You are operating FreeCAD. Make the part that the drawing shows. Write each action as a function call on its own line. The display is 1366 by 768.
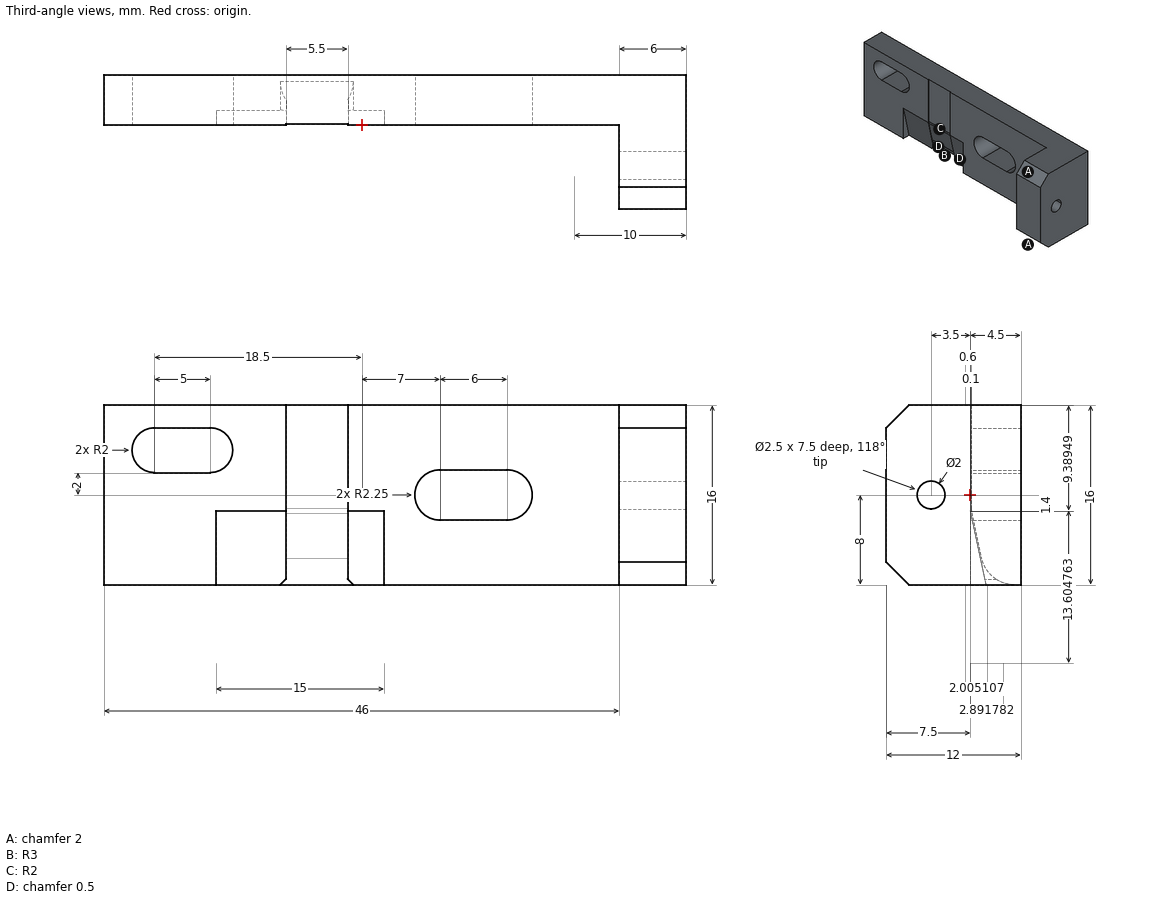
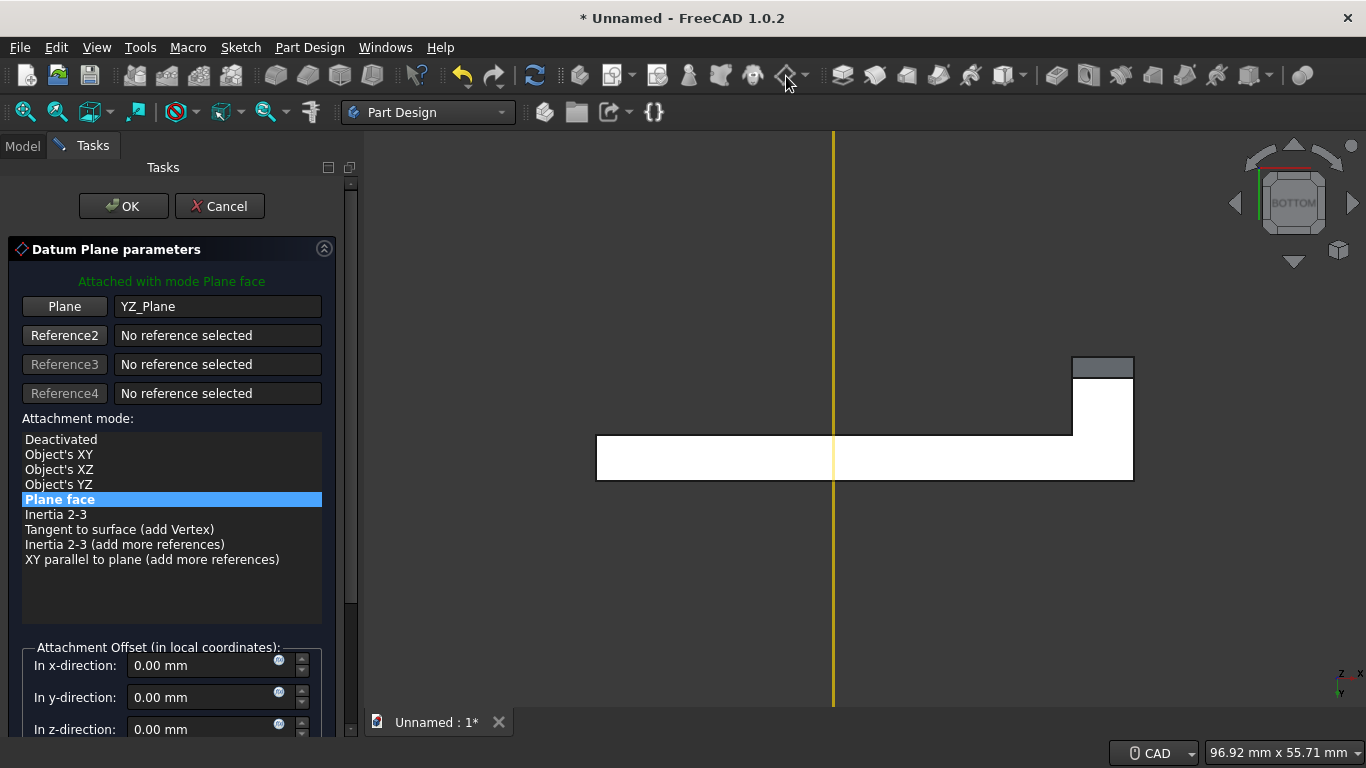
scroll(351, 456, down, 2)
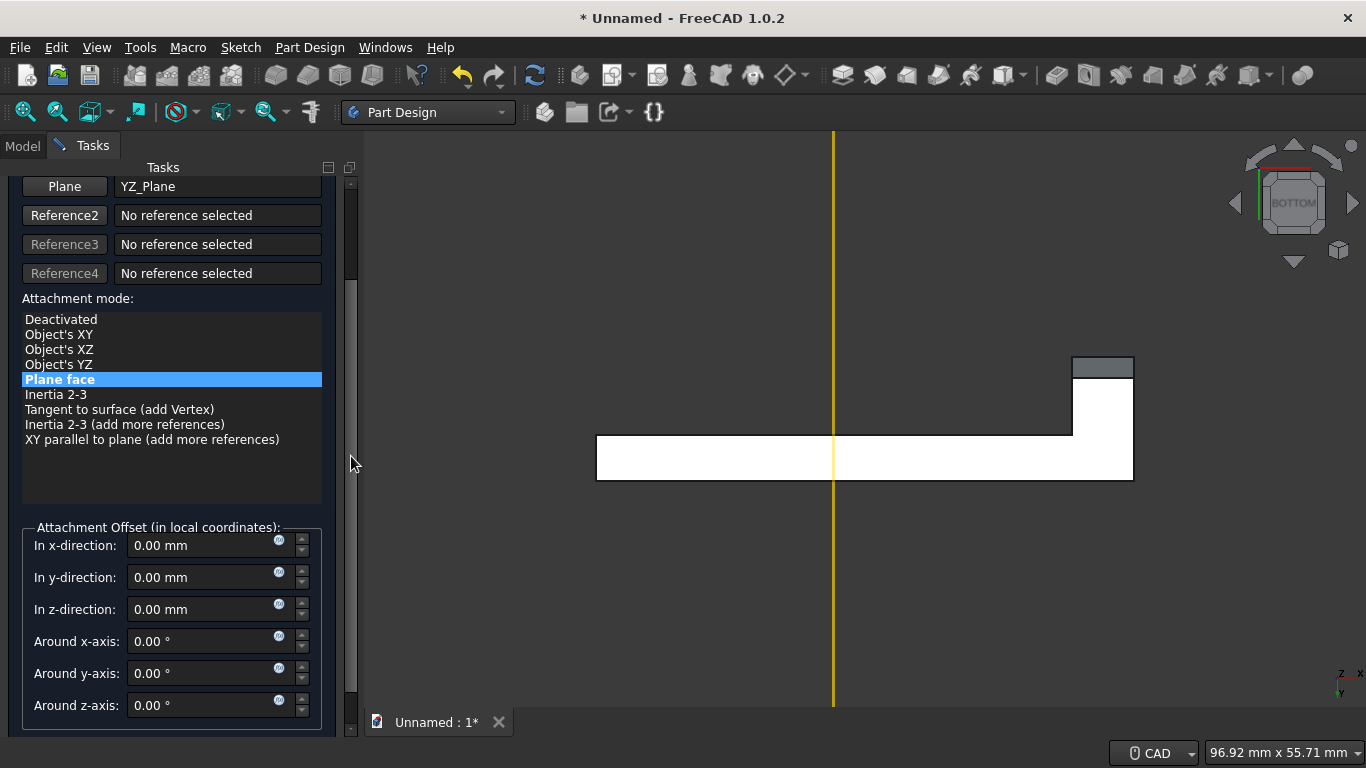
triple_click(210, 609)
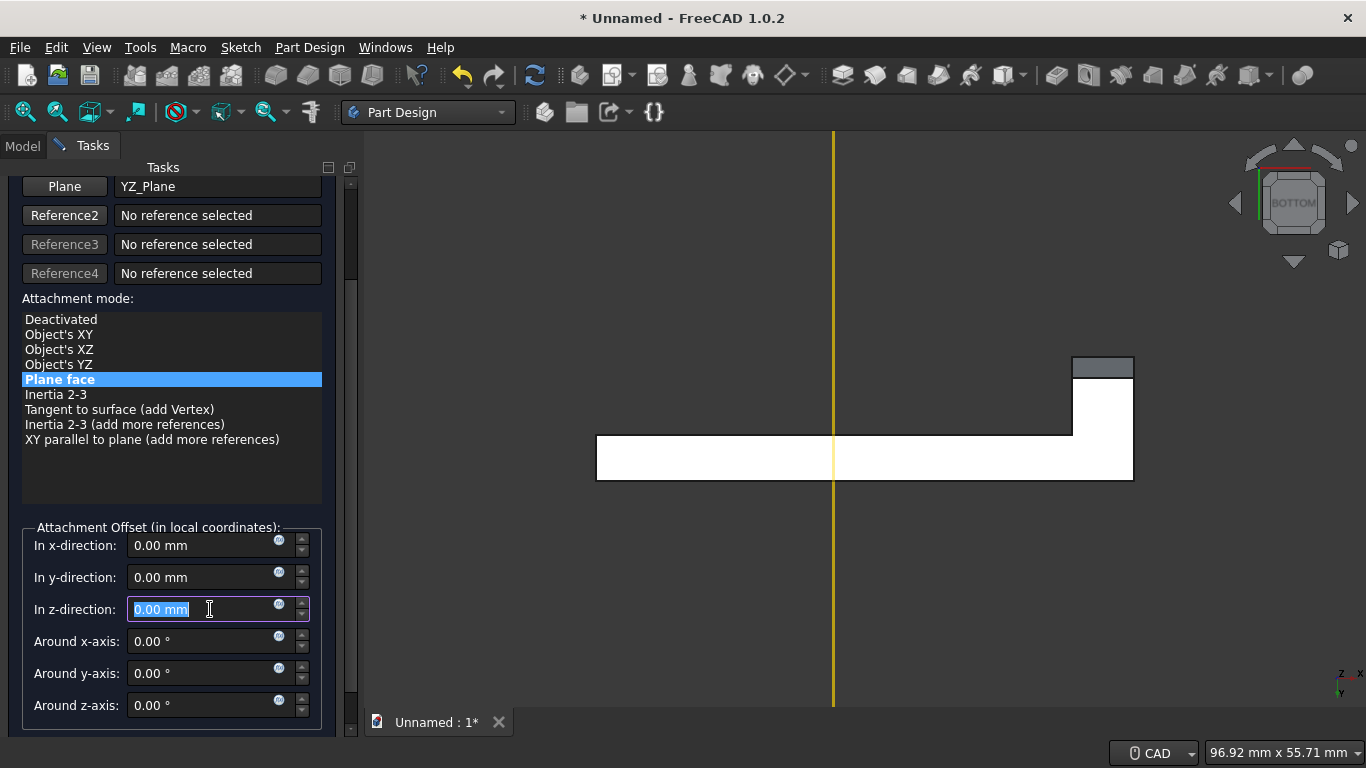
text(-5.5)
key(Tab)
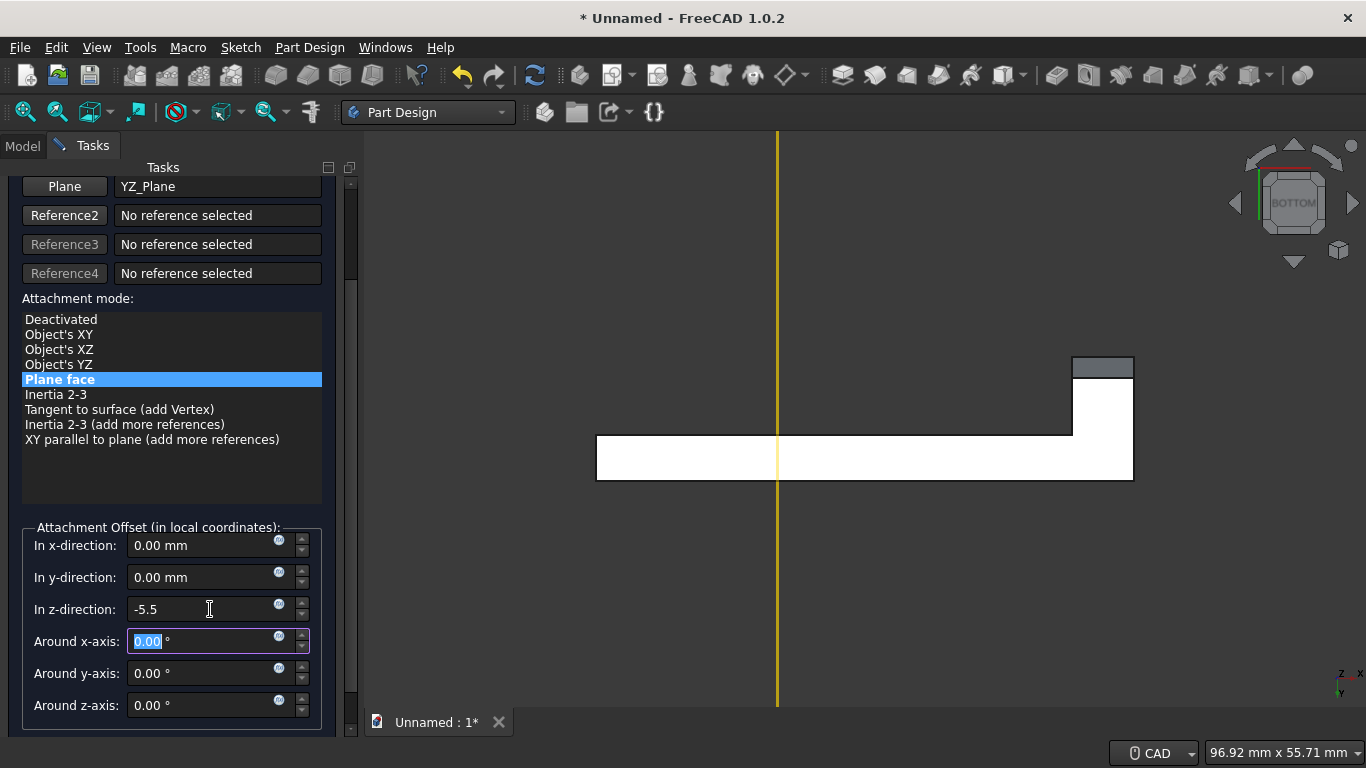
scroll(351, 456, up, 3)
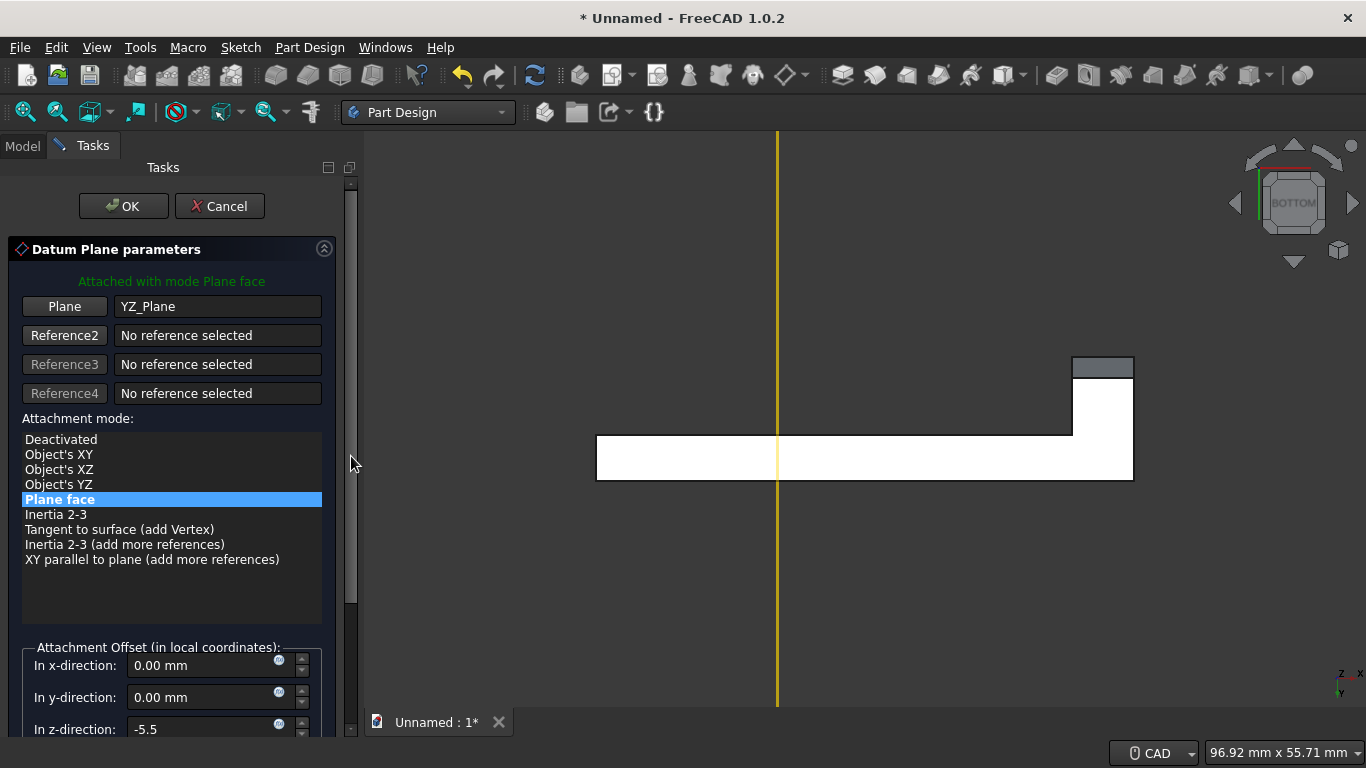
click(124, 206)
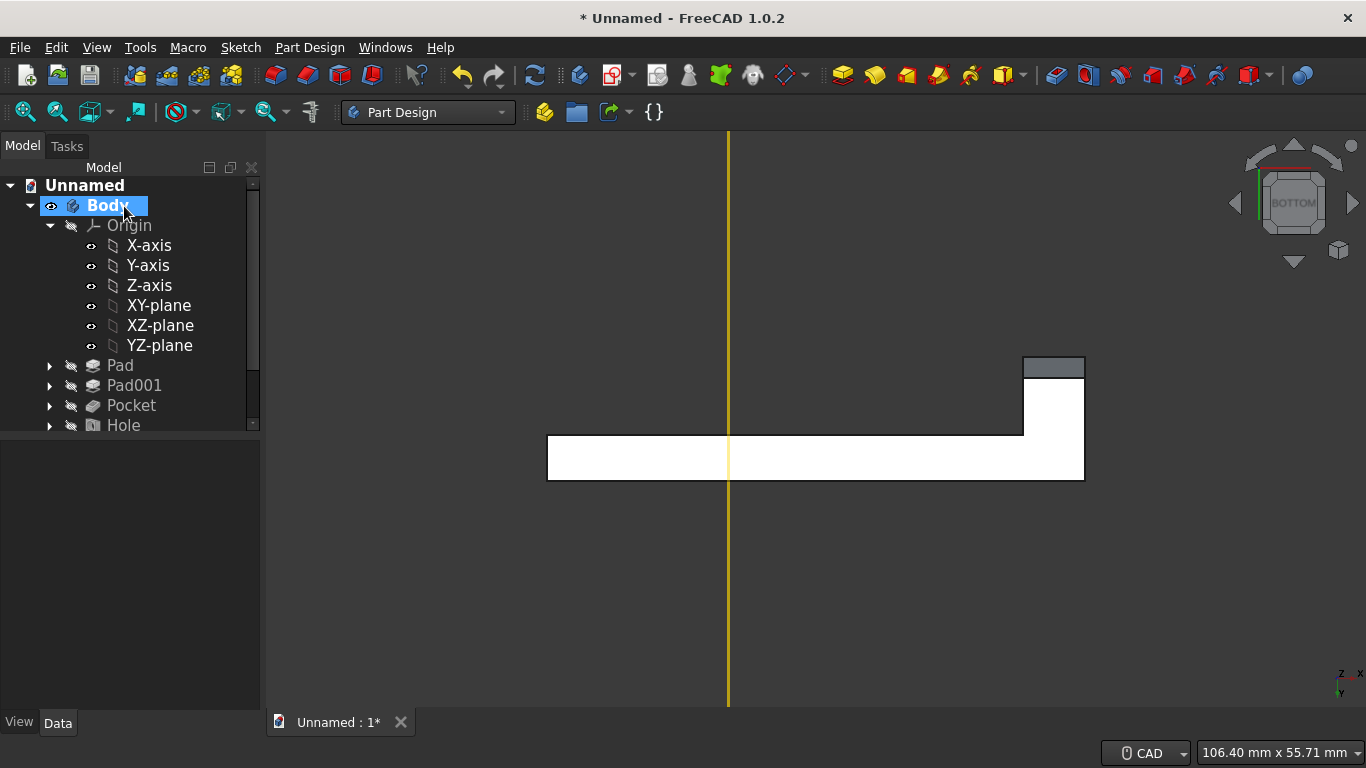
scroll(100, 301, down, 3)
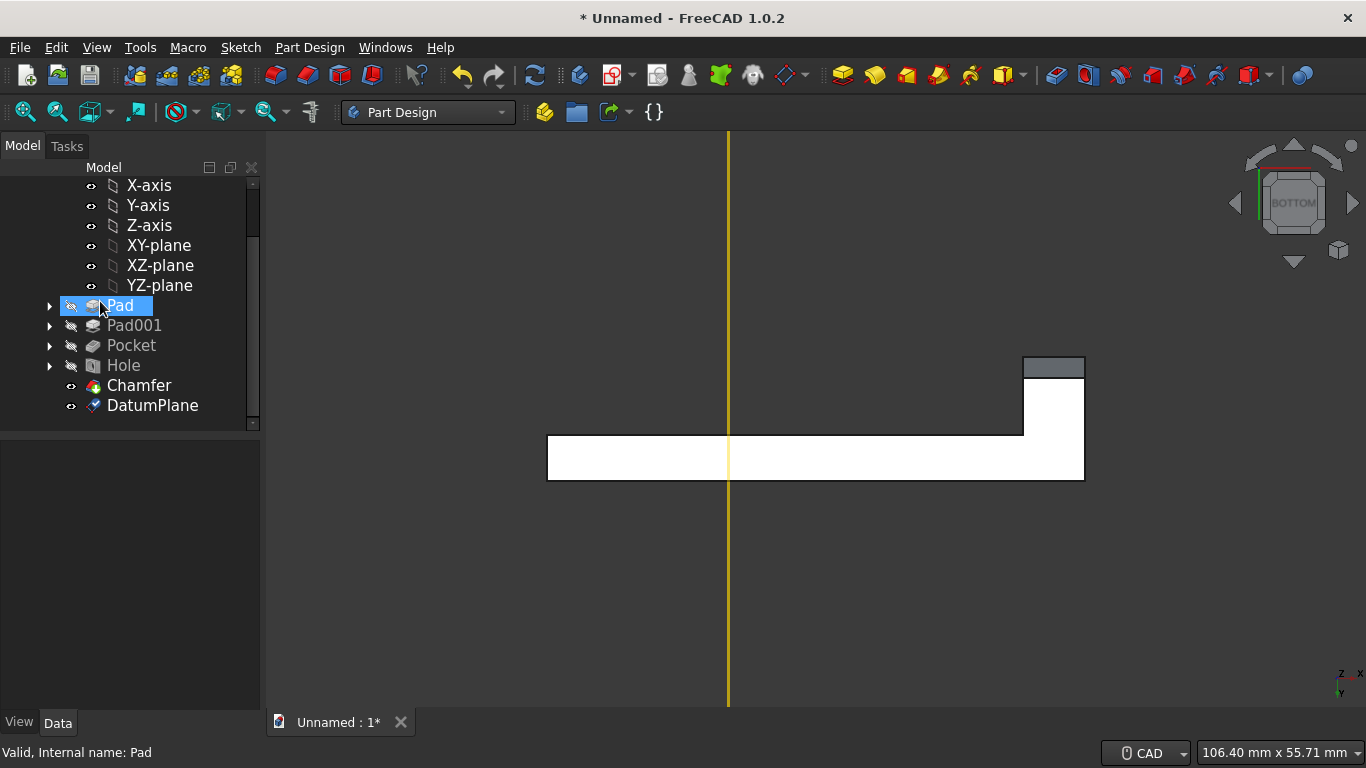
click(116, 406)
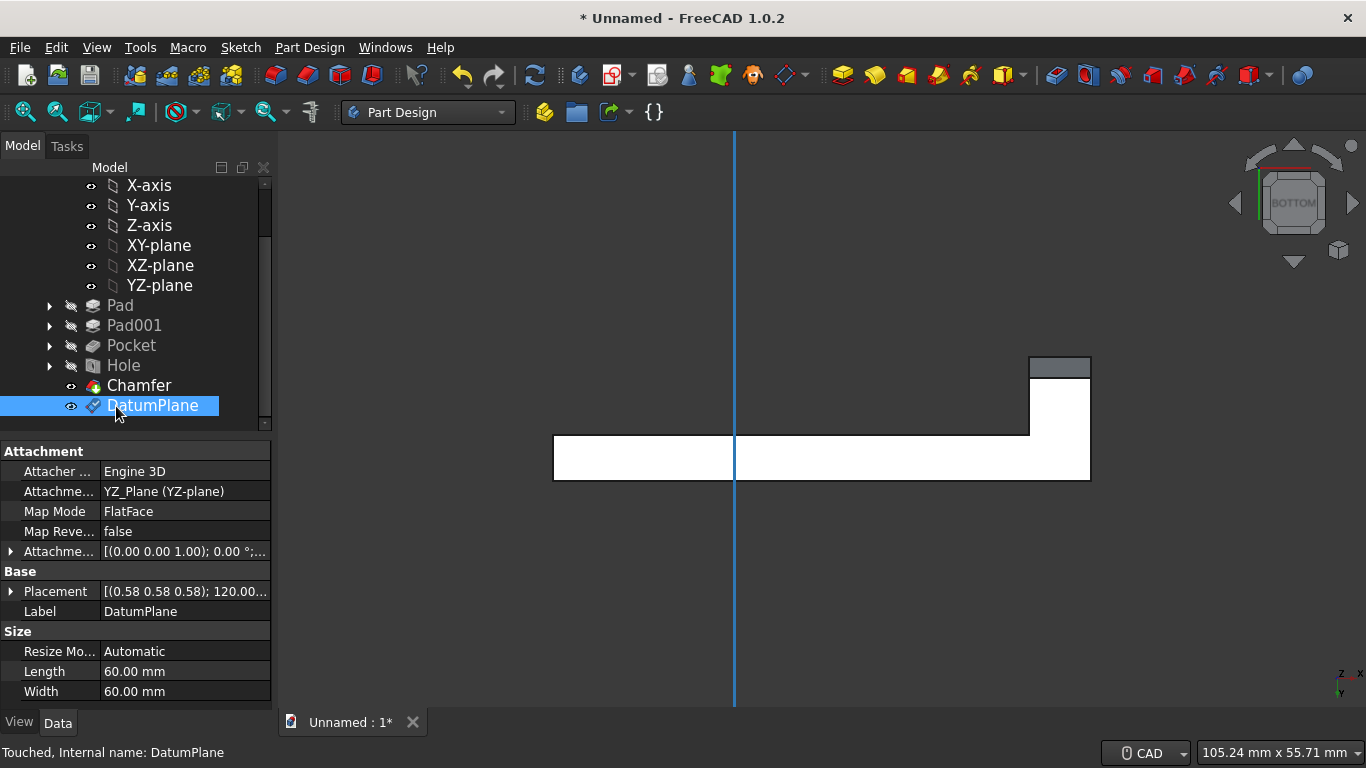
click(612, 76)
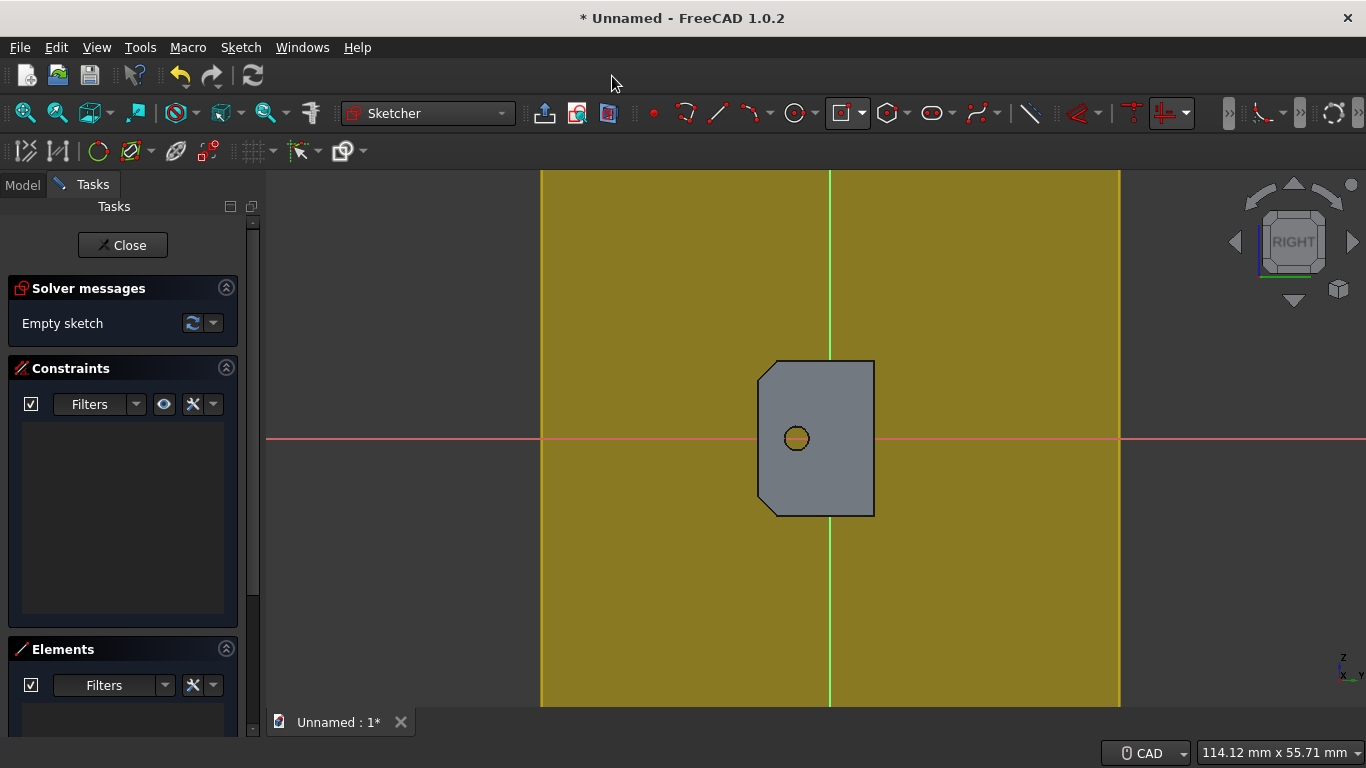
key(q)
key(s)